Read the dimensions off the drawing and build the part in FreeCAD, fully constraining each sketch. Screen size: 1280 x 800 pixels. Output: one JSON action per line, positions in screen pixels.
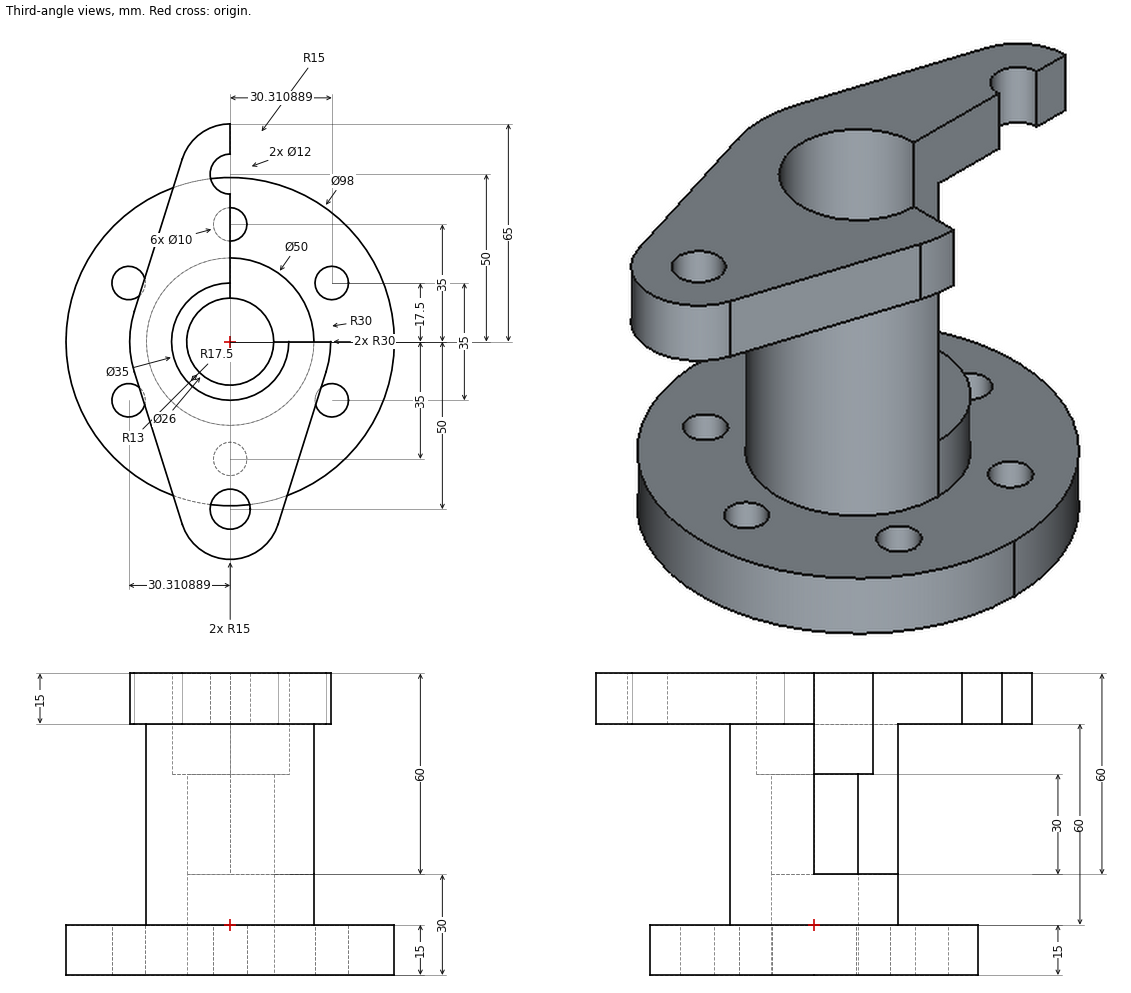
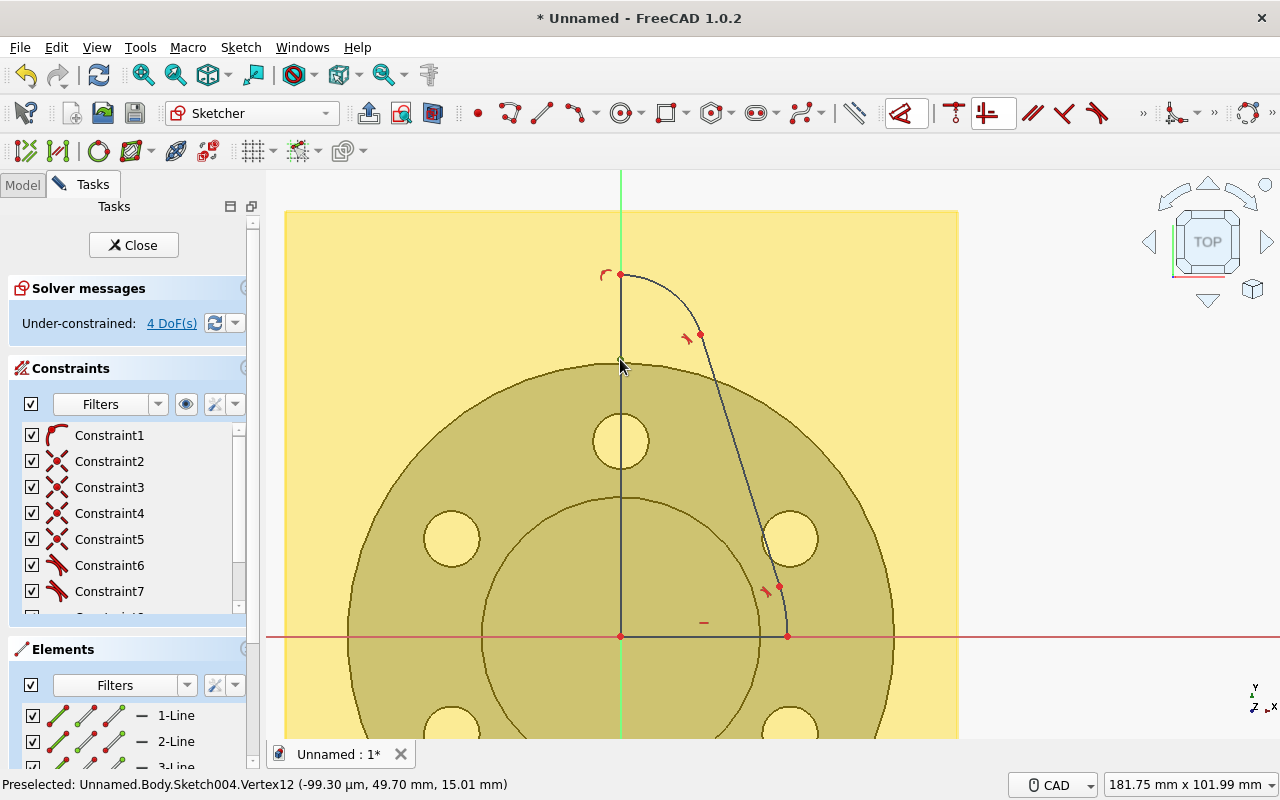
{"action": "left_click", "coordinate": [621, 674]}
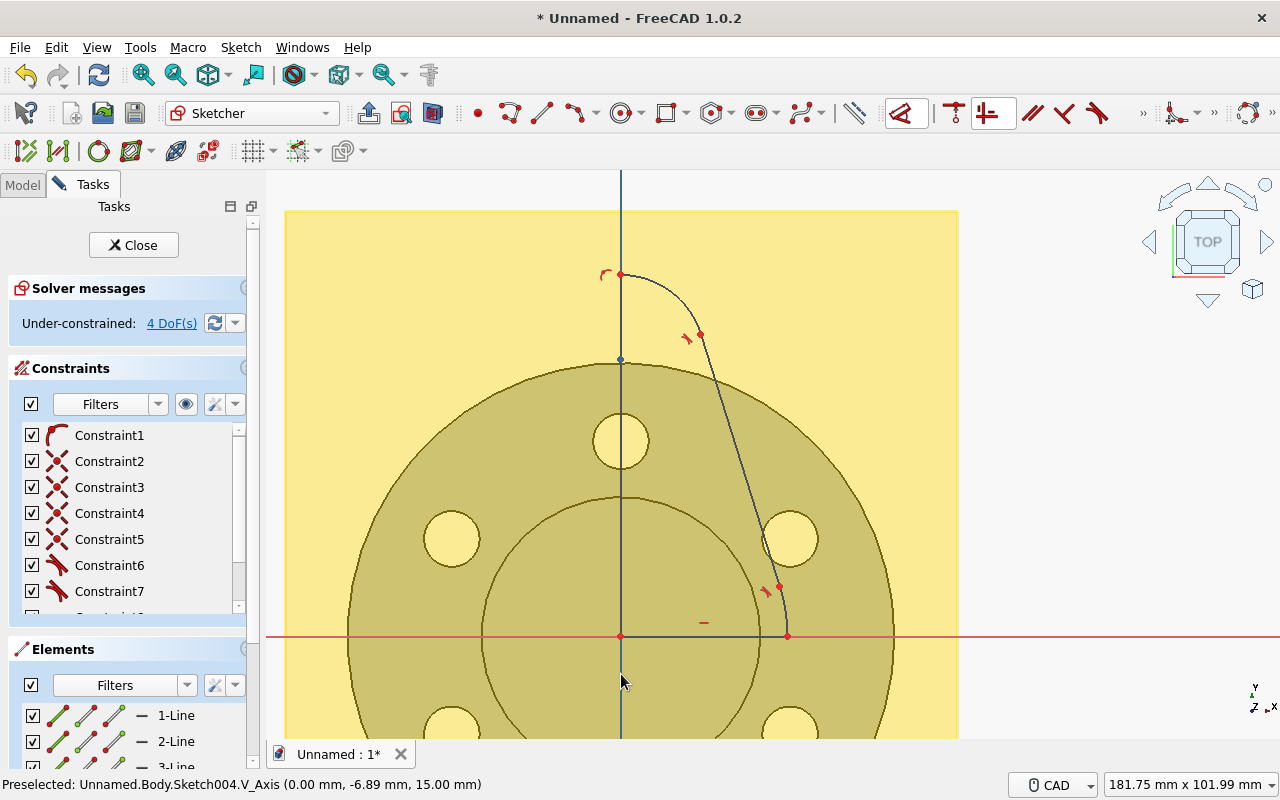
{"action": "key", "text": "c"}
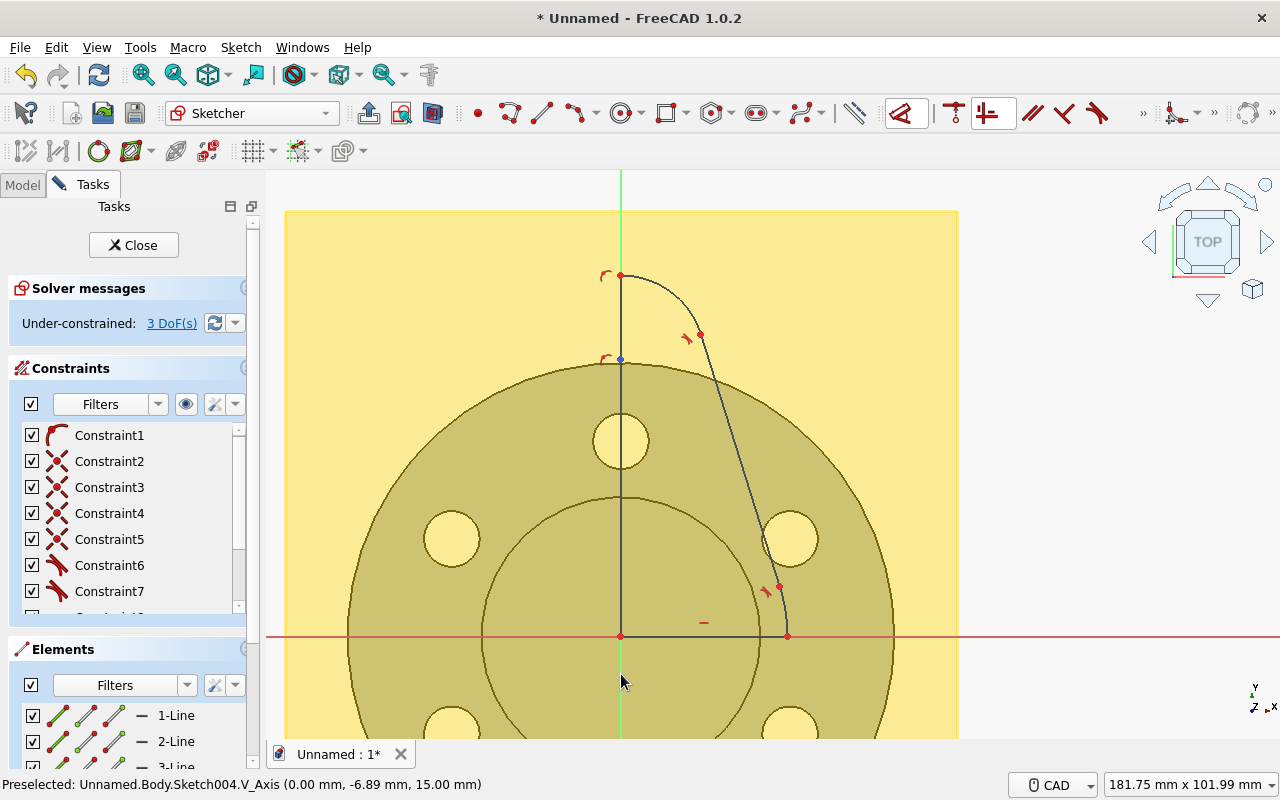
{"action": "left_click", "coordinate": [787, 621]}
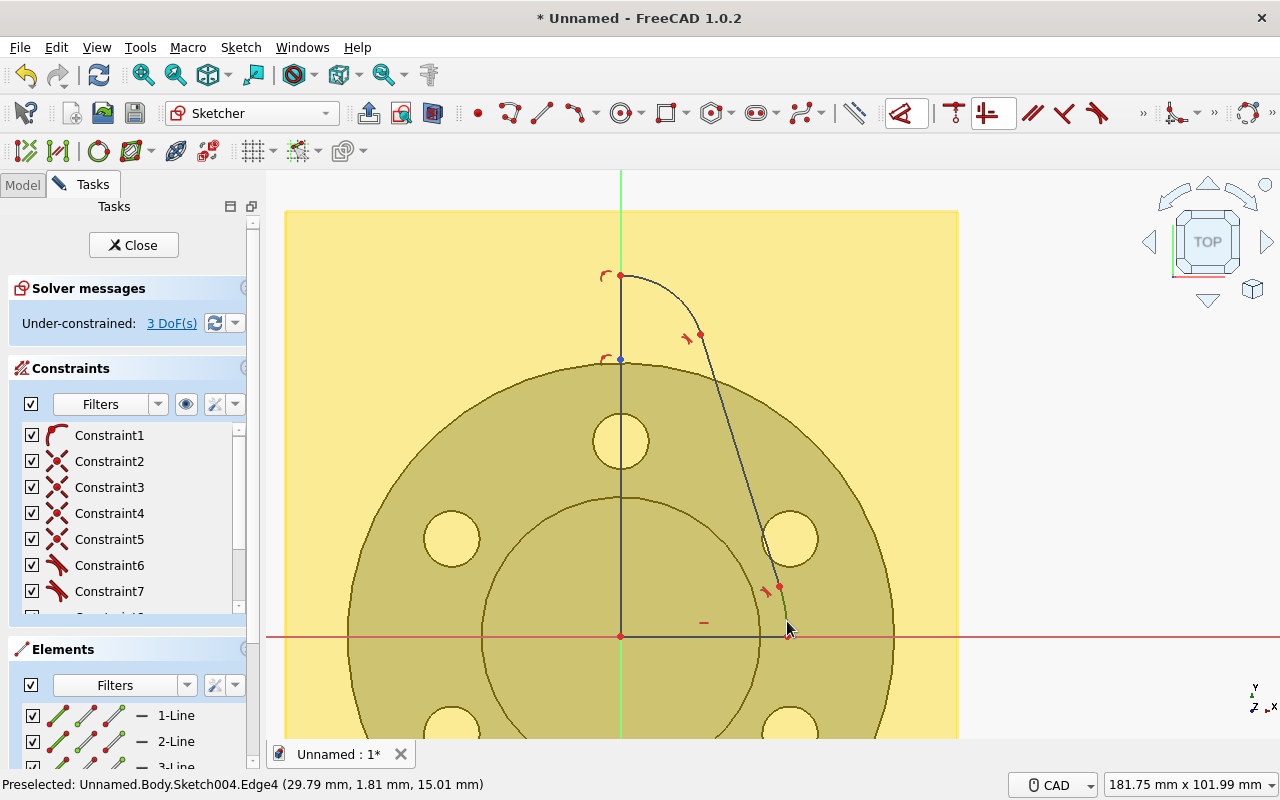
{"action": "key", "text": "k r"}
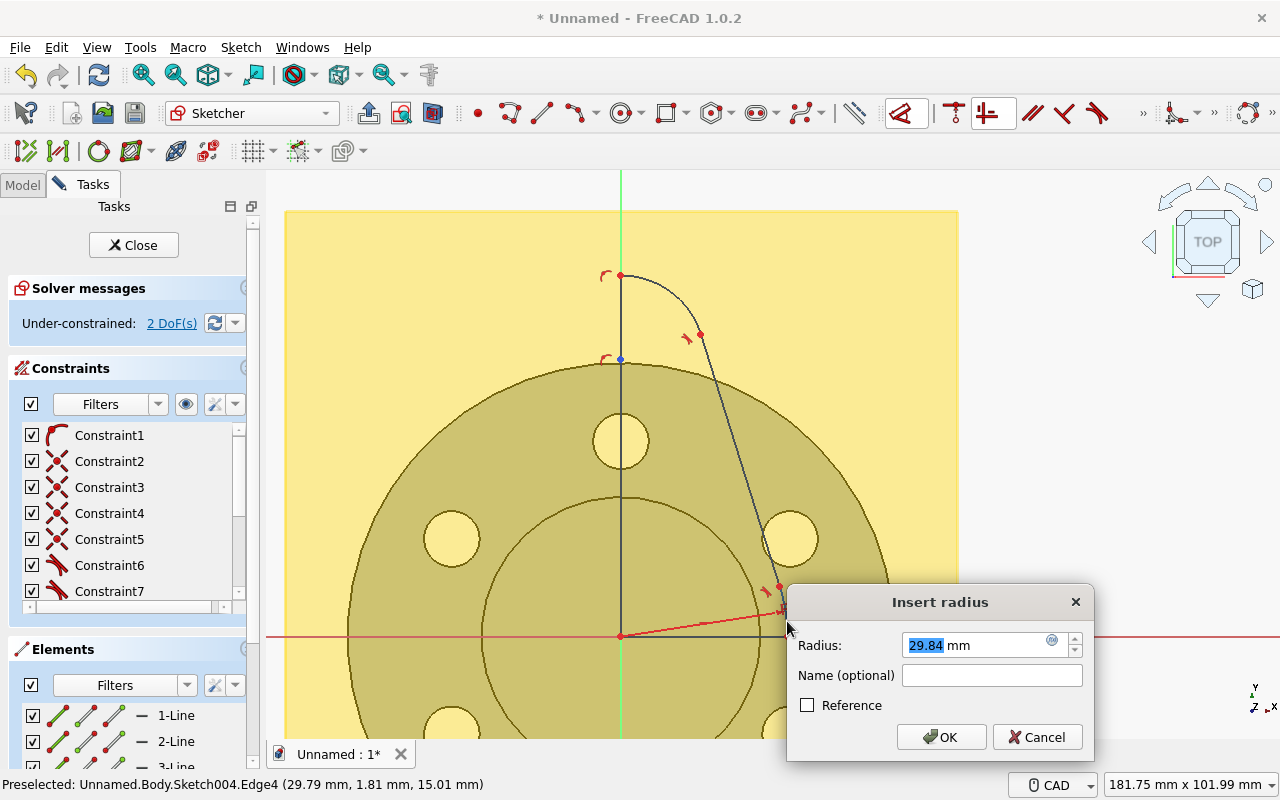
{"action": "type", "text": "30"}
{"action": "key", "text": "Return"}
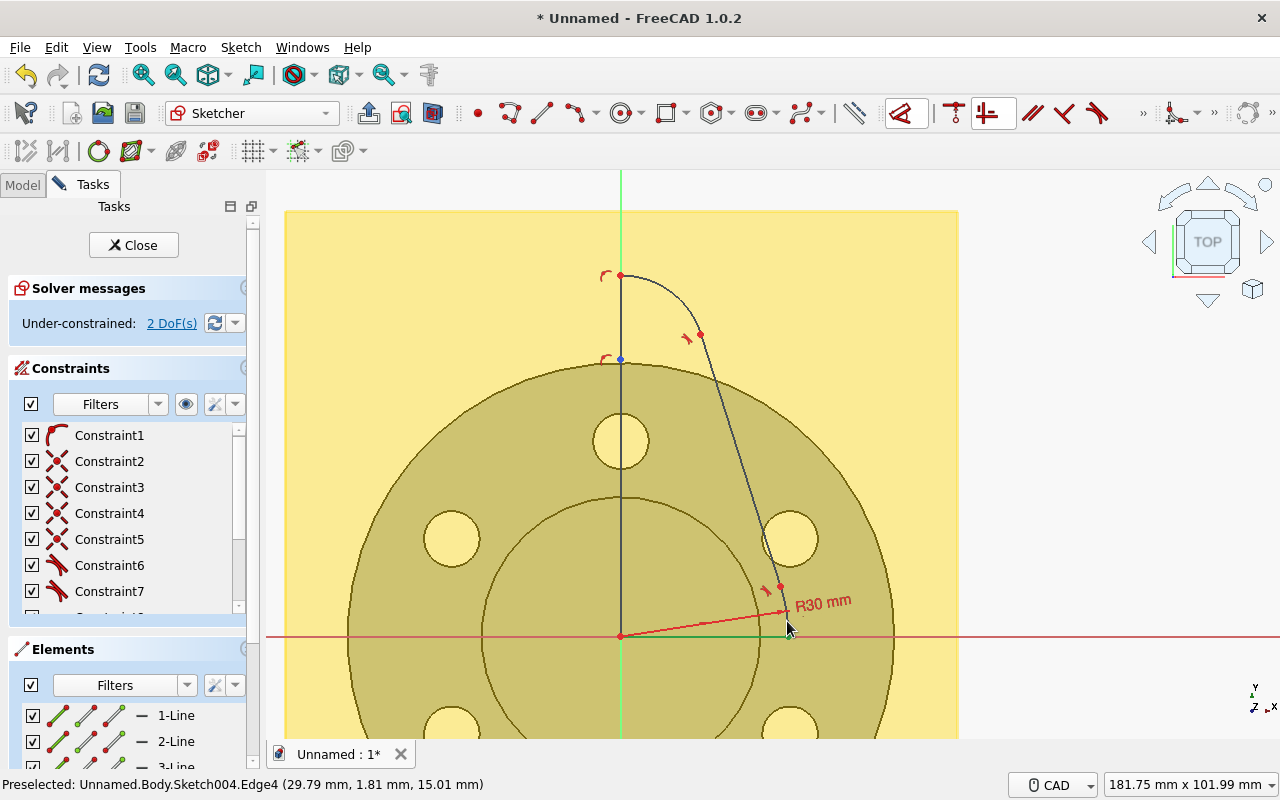
{"action": "left_click", "coordinate": [686, 306]}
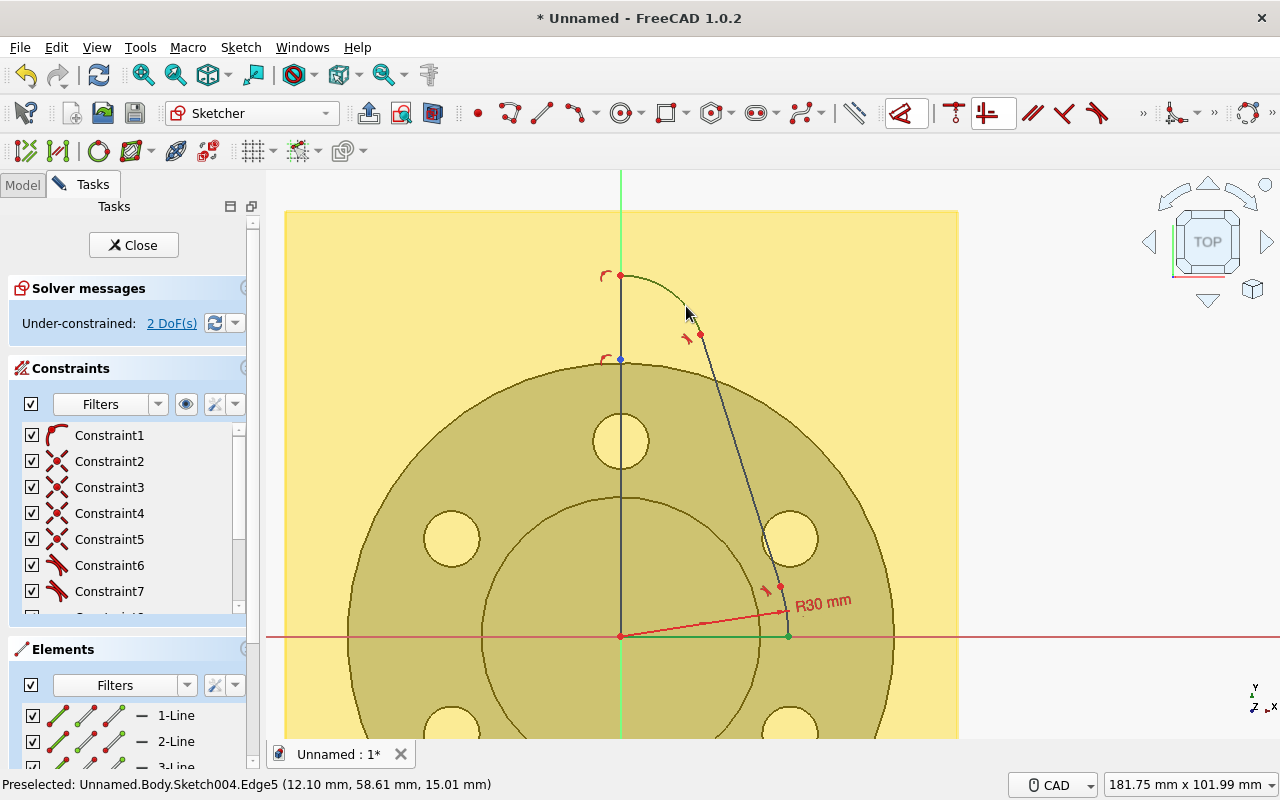
{"action": "key", "text": "k r"}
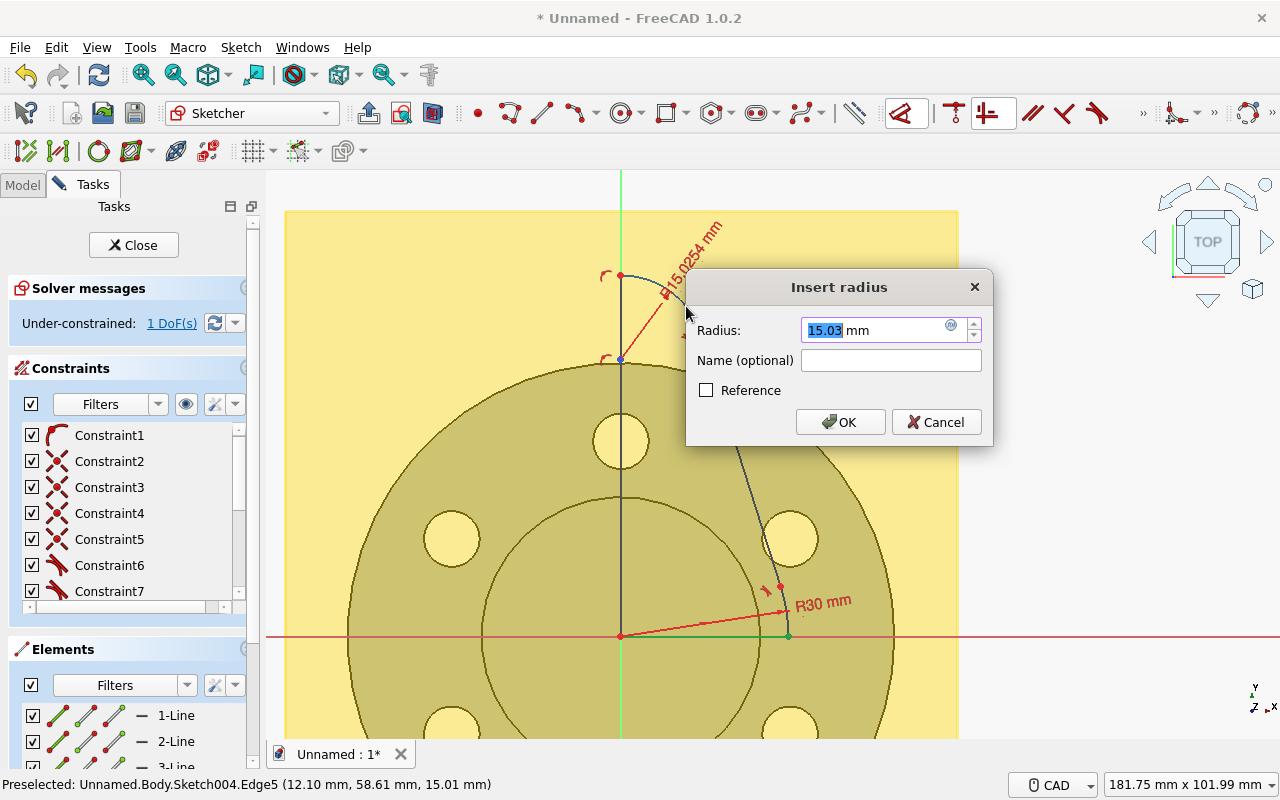
{"action": "type", "text": "15"}
{"action": "key", "text": "Return"}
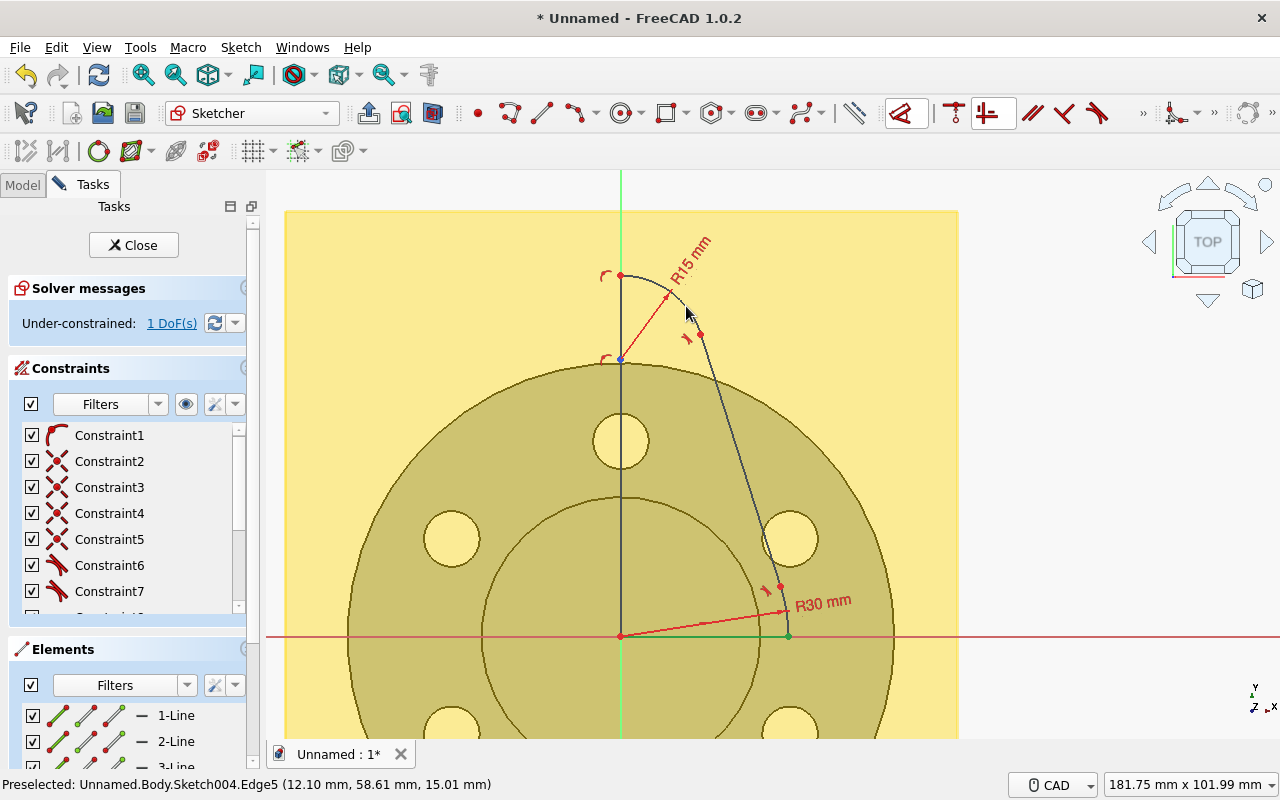
{"action": "left_click", "coordinate": [621, 384]}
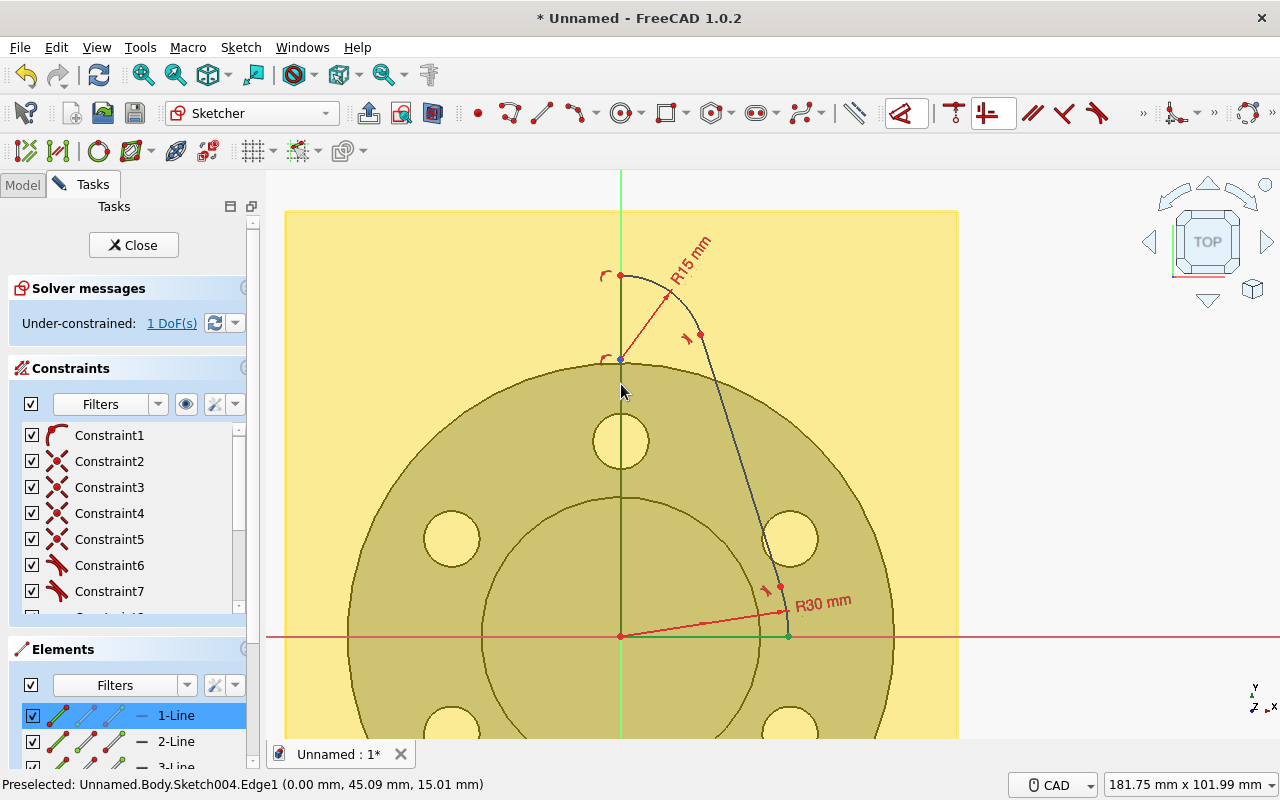
{"action": "left_click", "coordinate": [922, 114]}